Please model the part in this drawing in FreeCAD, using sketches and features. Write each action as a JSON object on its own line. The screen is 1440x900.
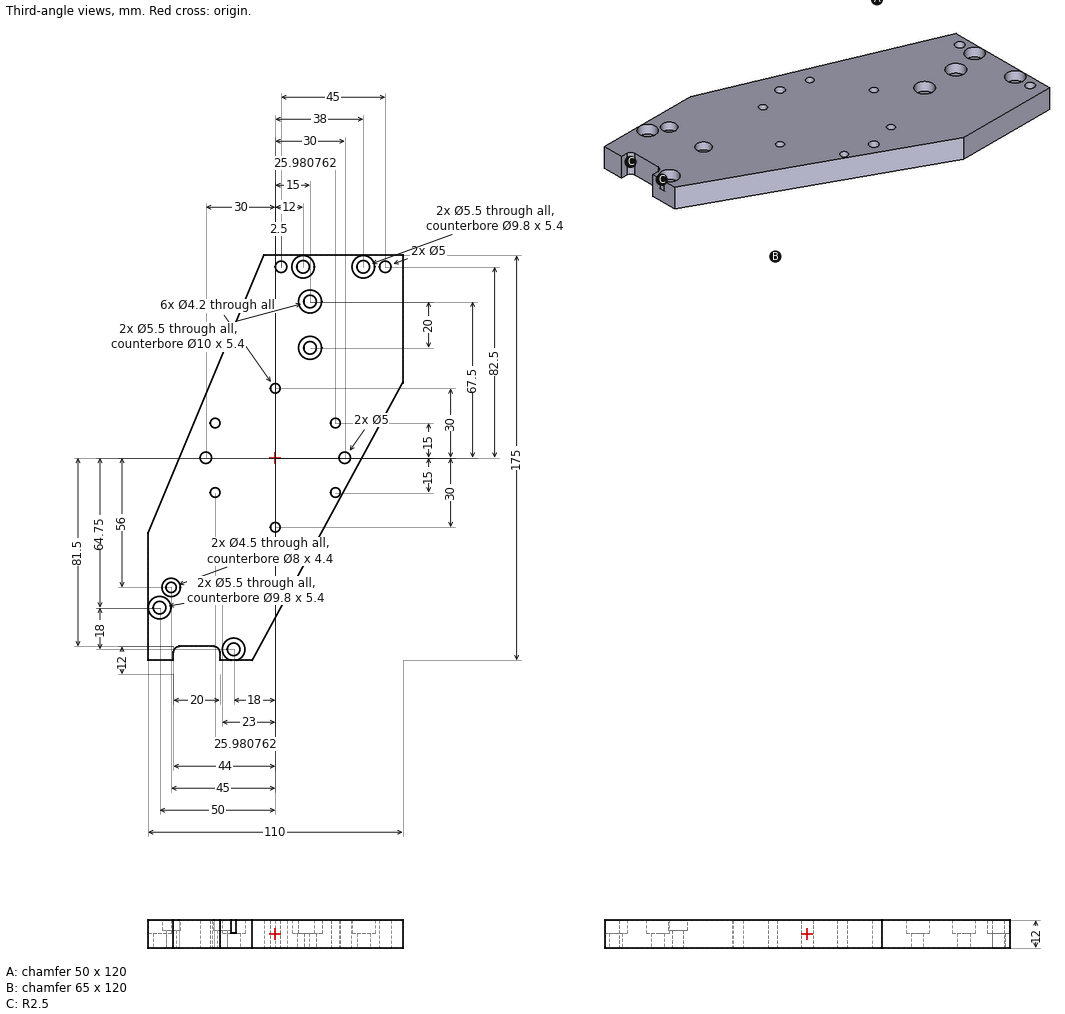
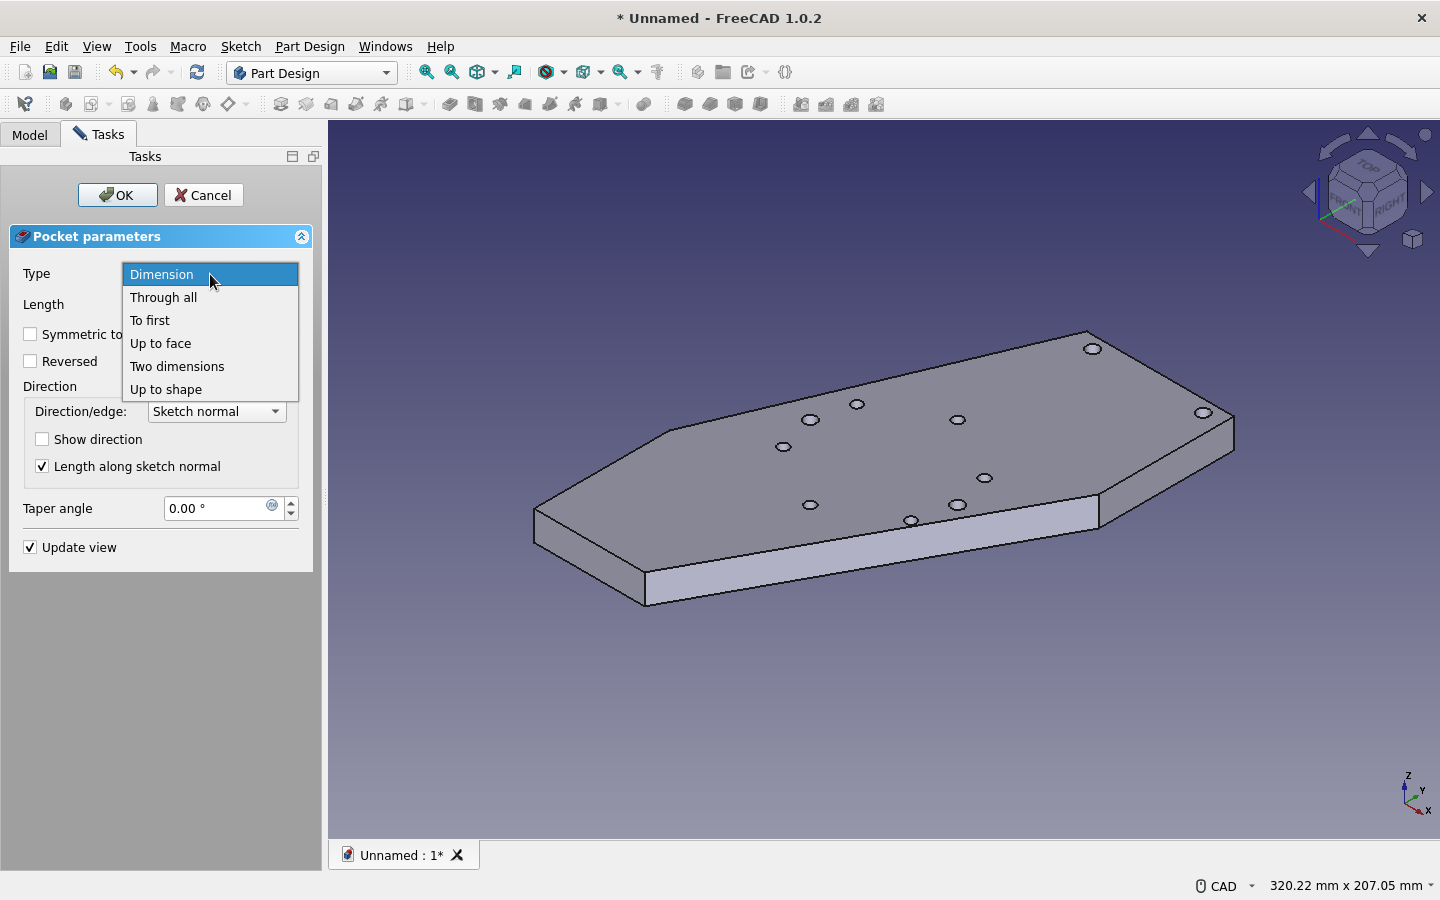
{"action": "left_click", "coordinate": [208, 298]}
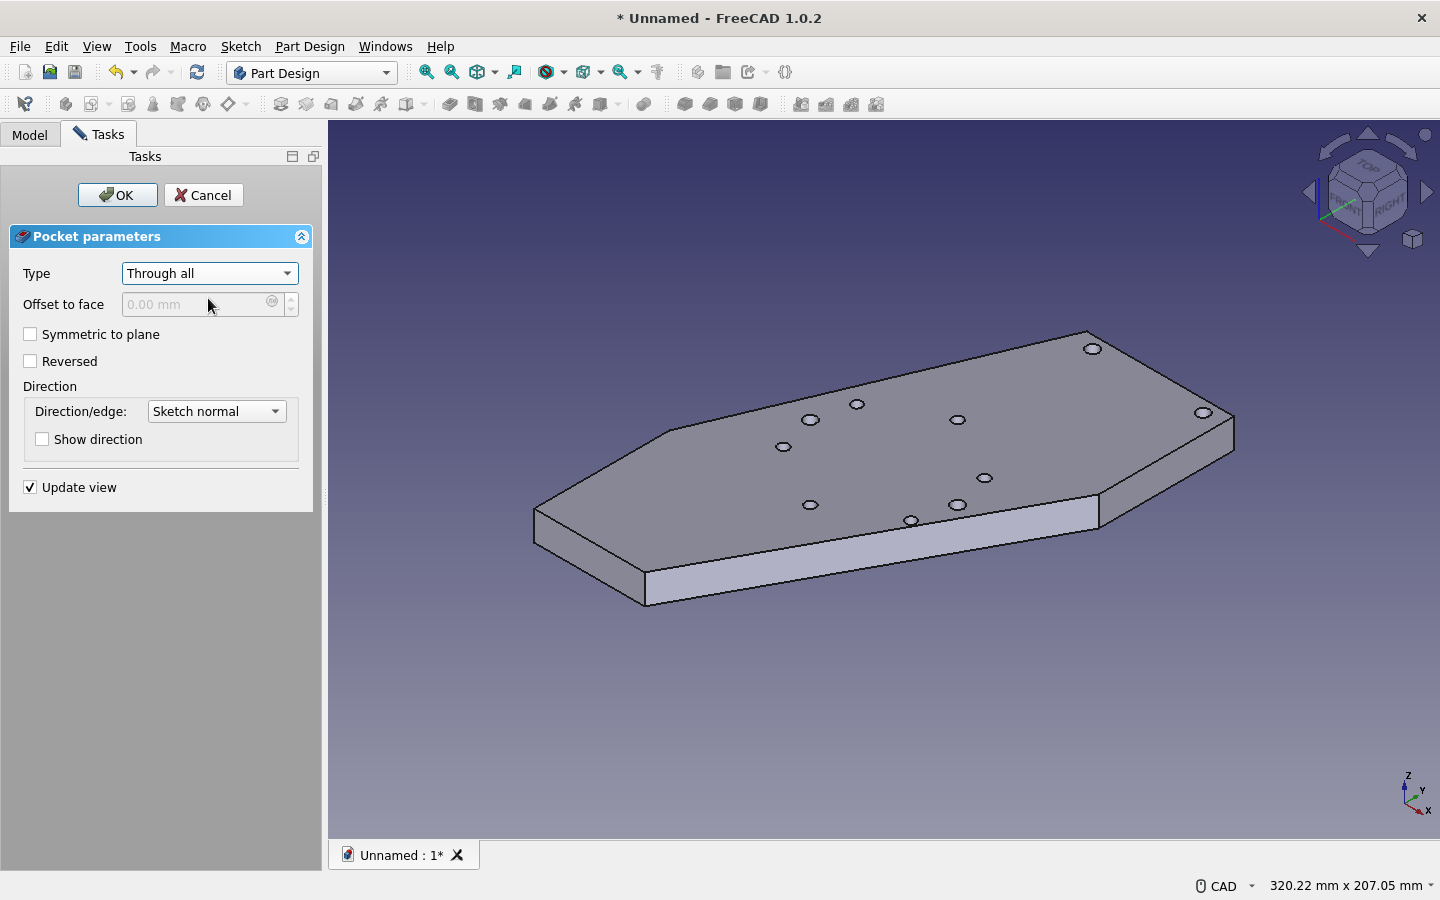
{"action": "left_click", "coordinate": [118, 195]}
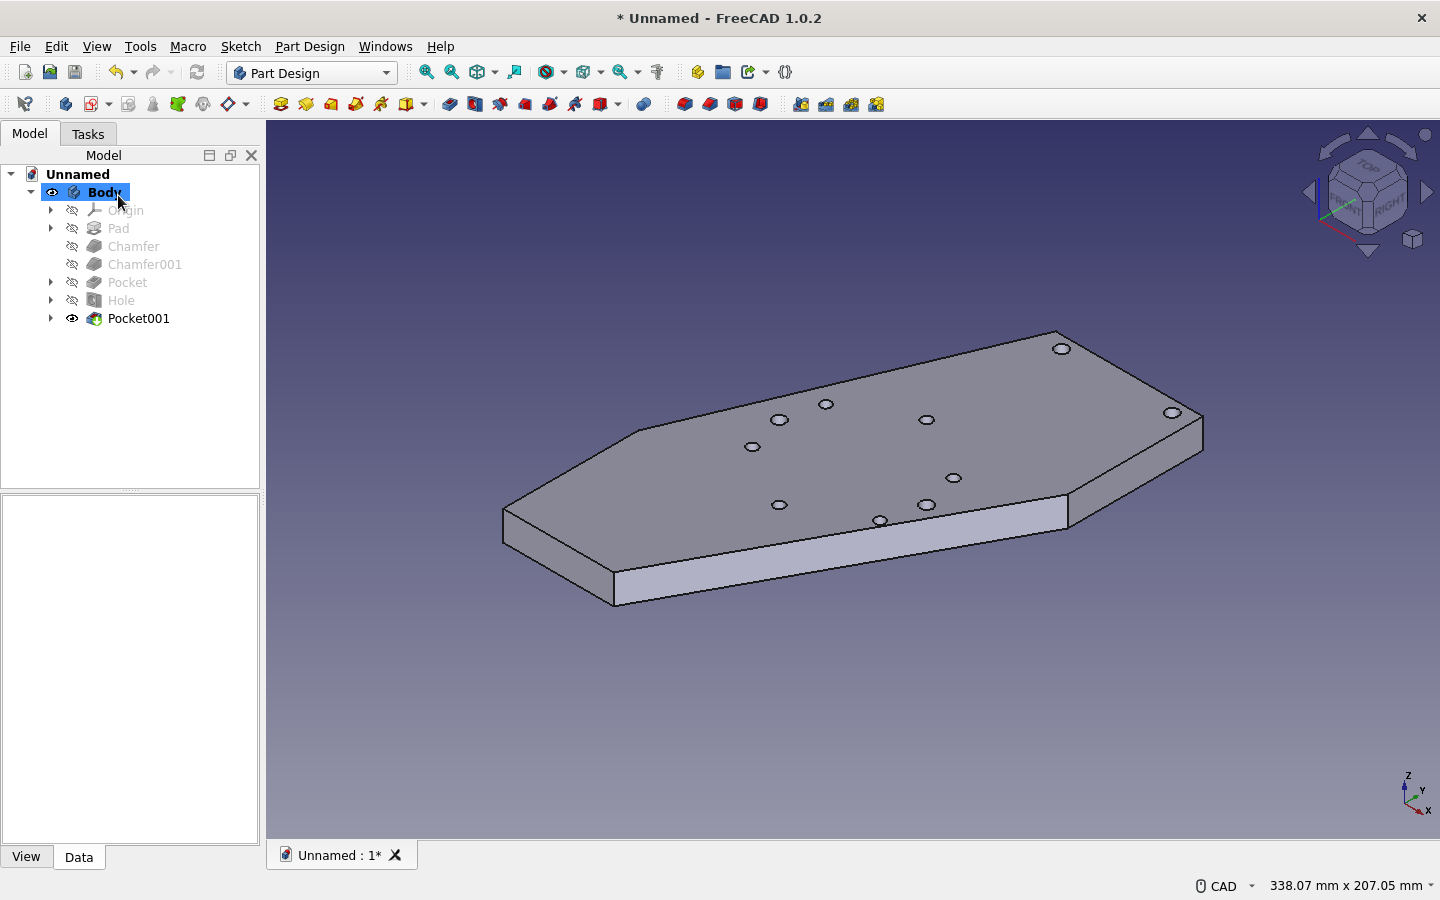
{"action": "left_click", "coordinate": [853, 461]}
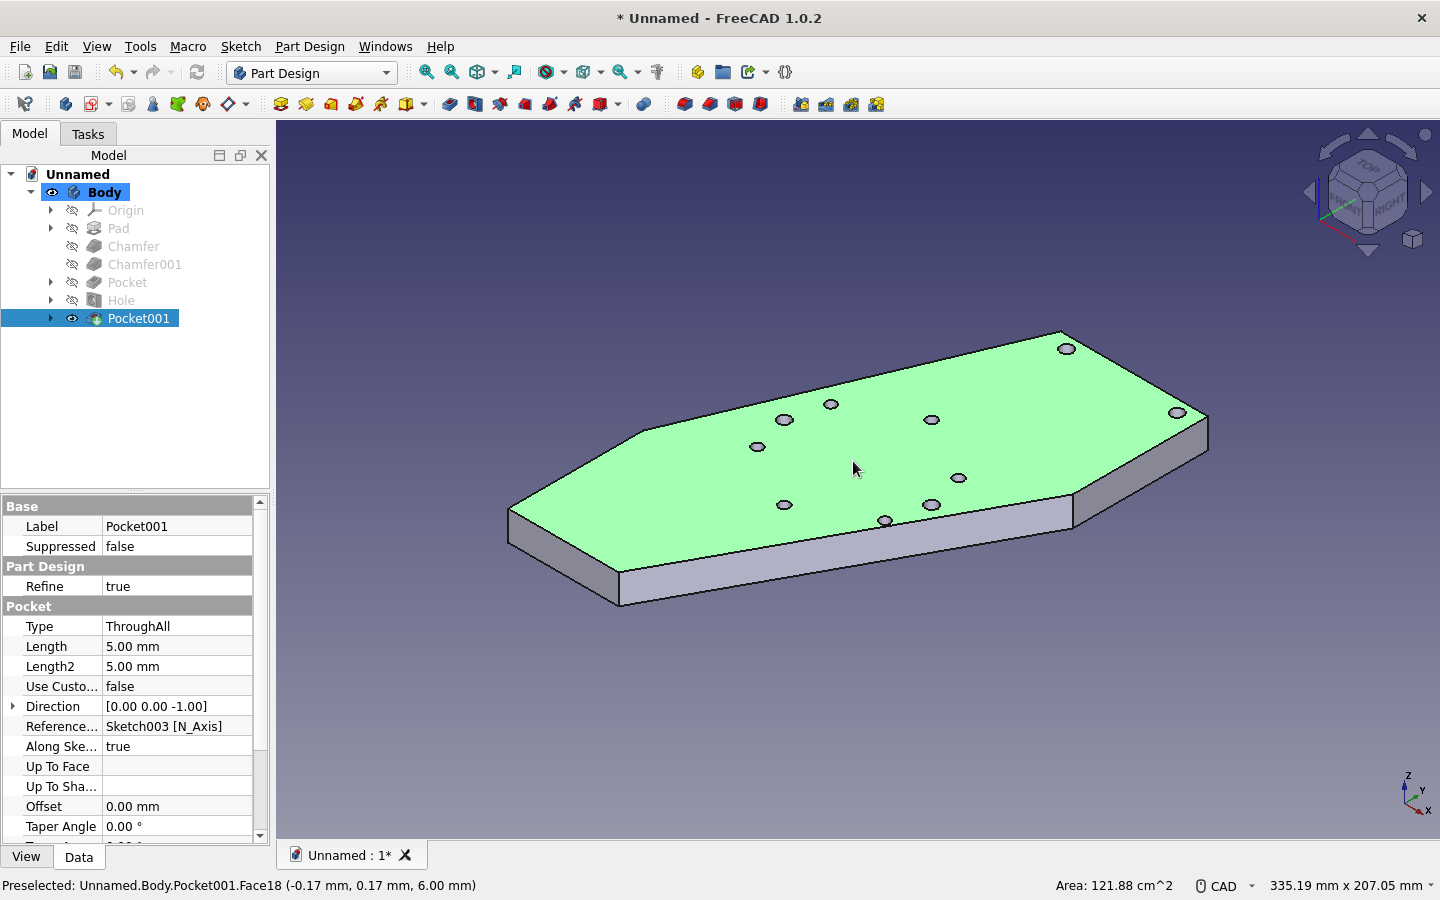
{"action": "left_click", "coordinate": [90, 104]}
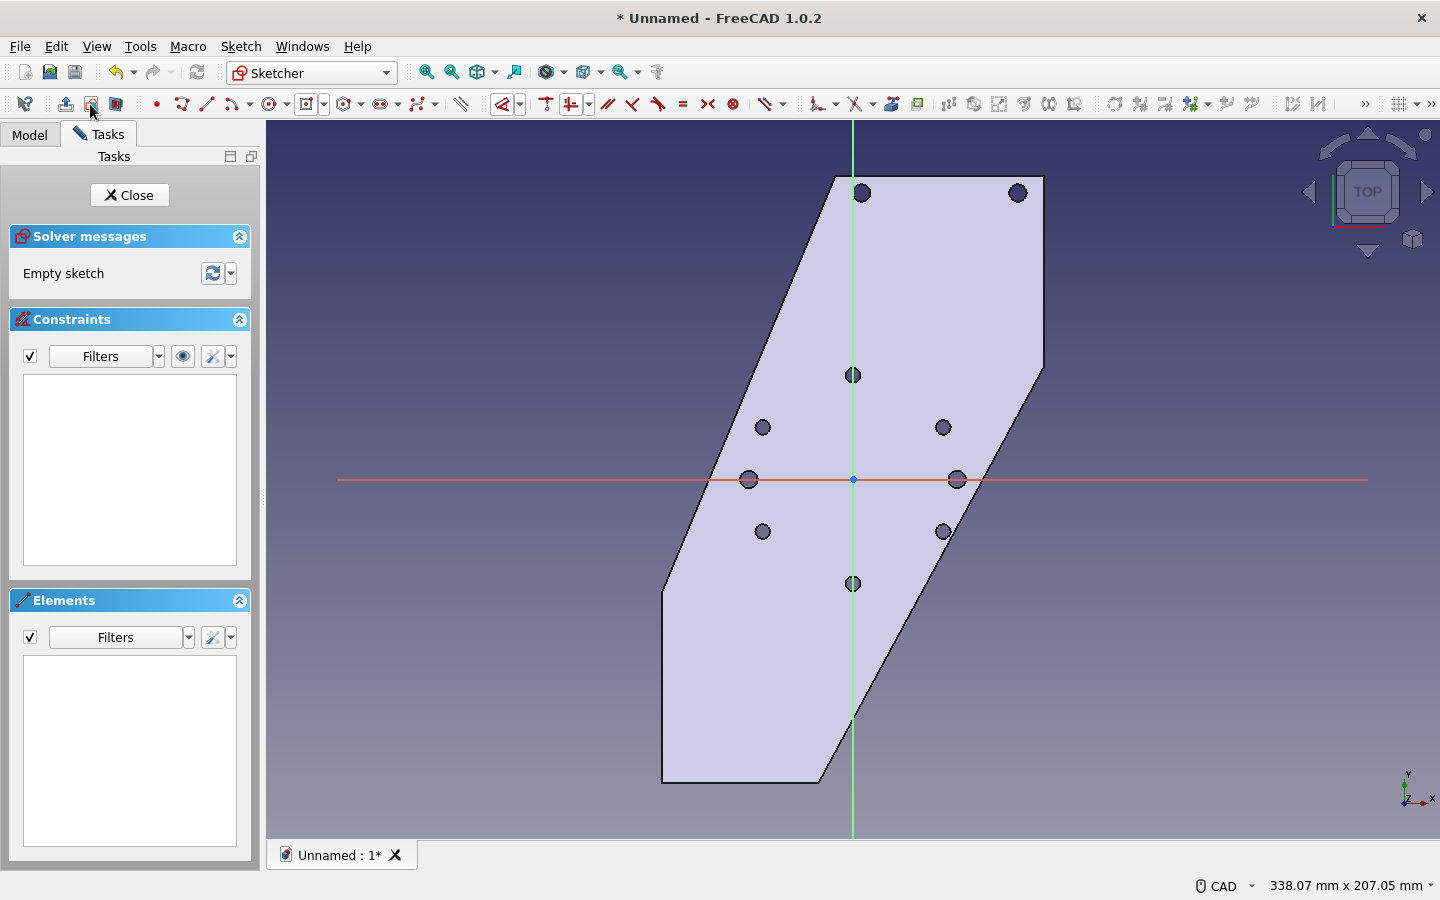
{"action": "scroll", "coordinate": [971, 148], "scroll_direction": "up", "scroll_amount": 9}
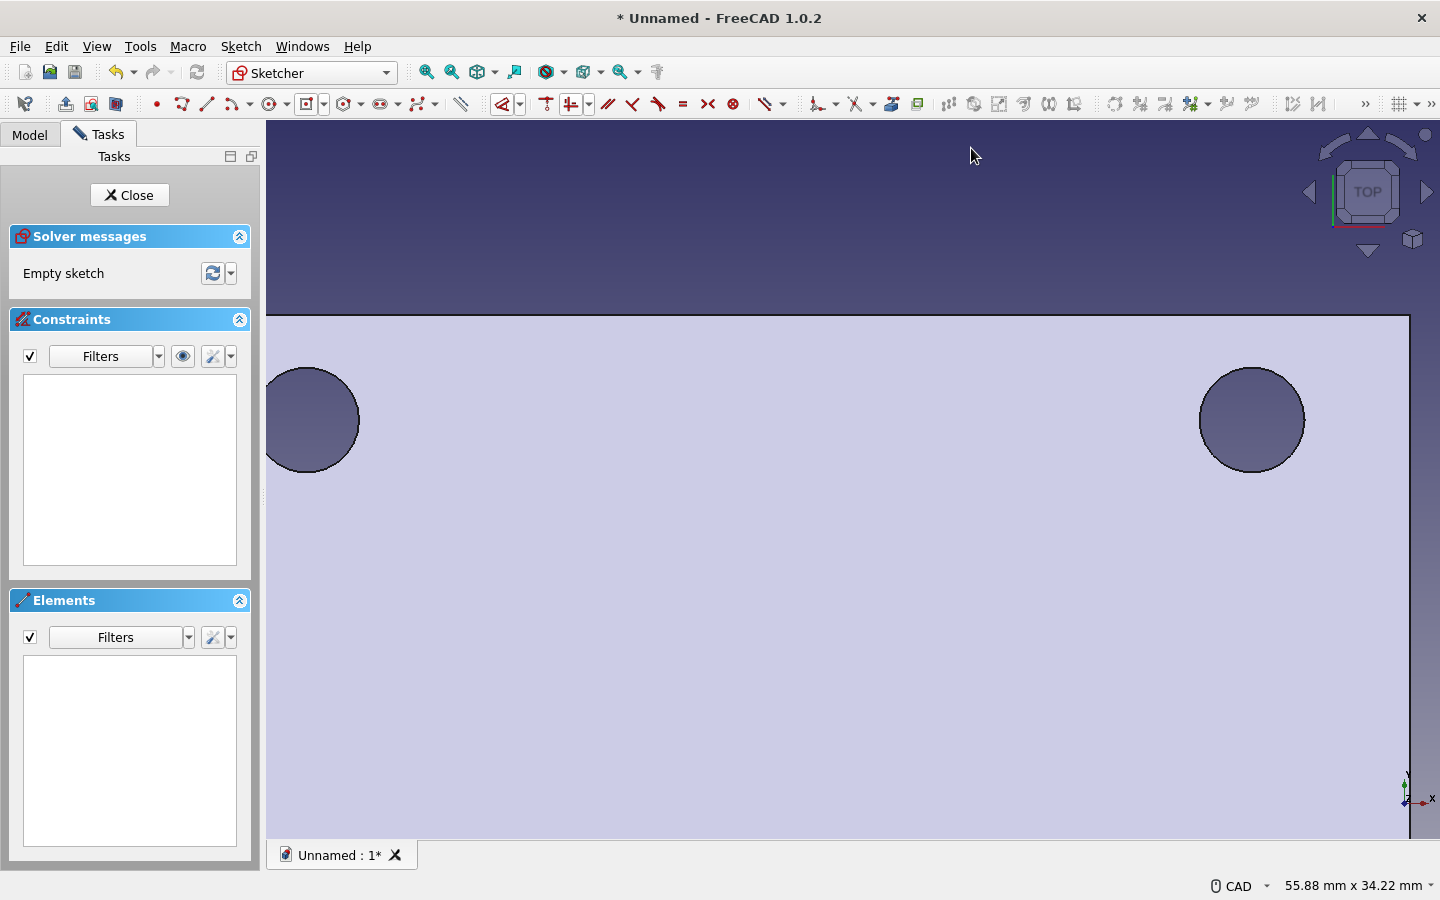
{"action": "key", "text": "g c"}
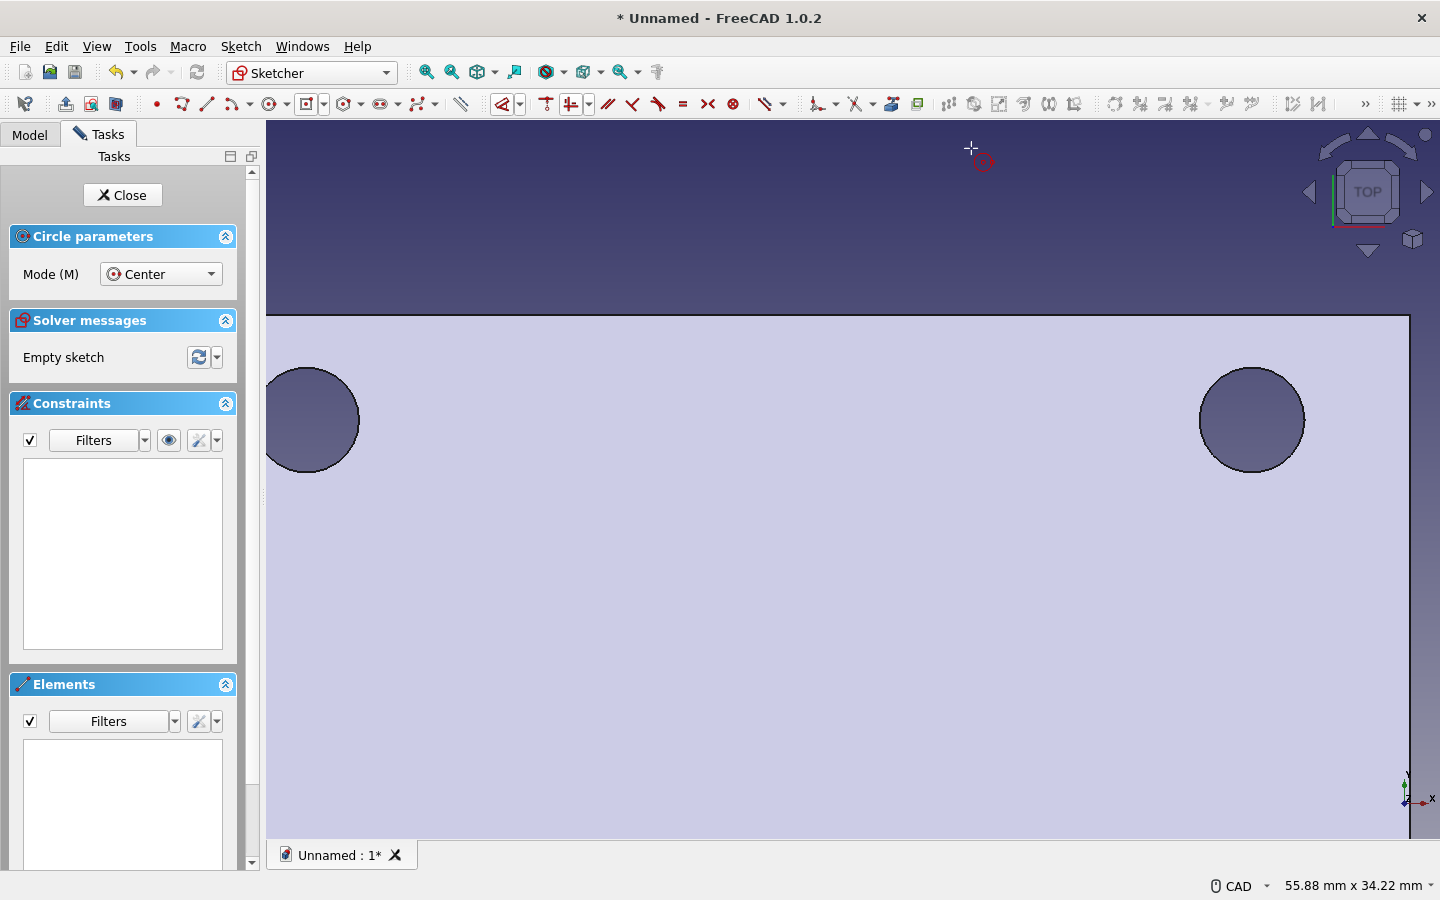
{"action": "left_click", "coordinate": [1052, 420]}
{"action": "left_click", "coordinate": [1093, 379]}